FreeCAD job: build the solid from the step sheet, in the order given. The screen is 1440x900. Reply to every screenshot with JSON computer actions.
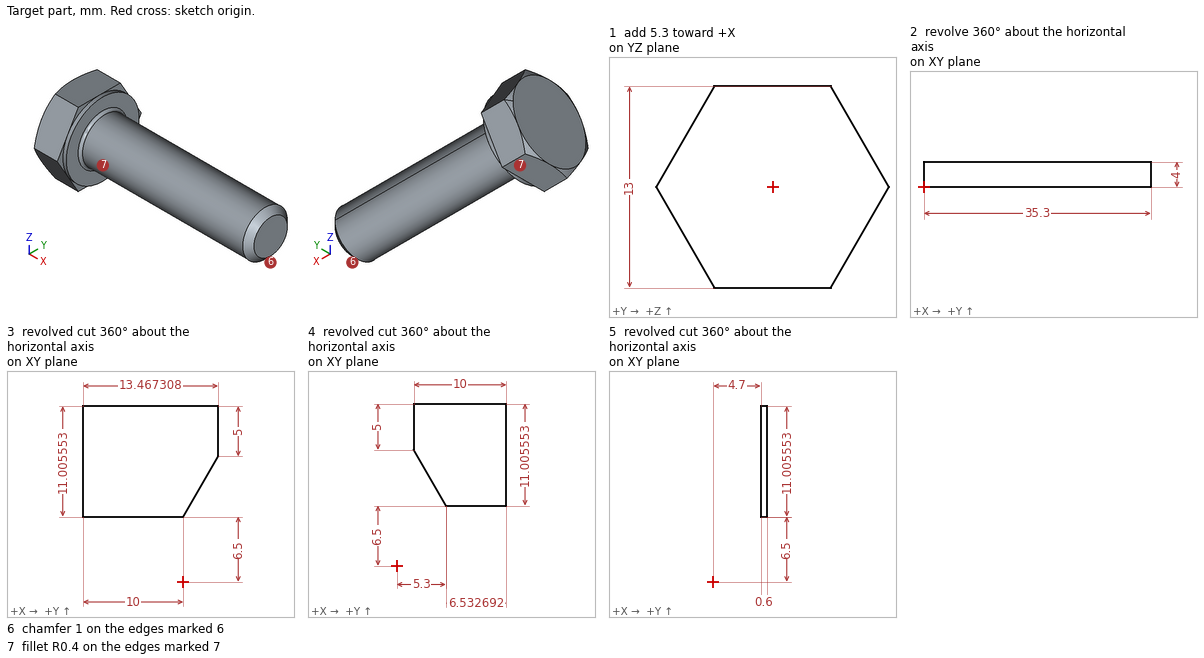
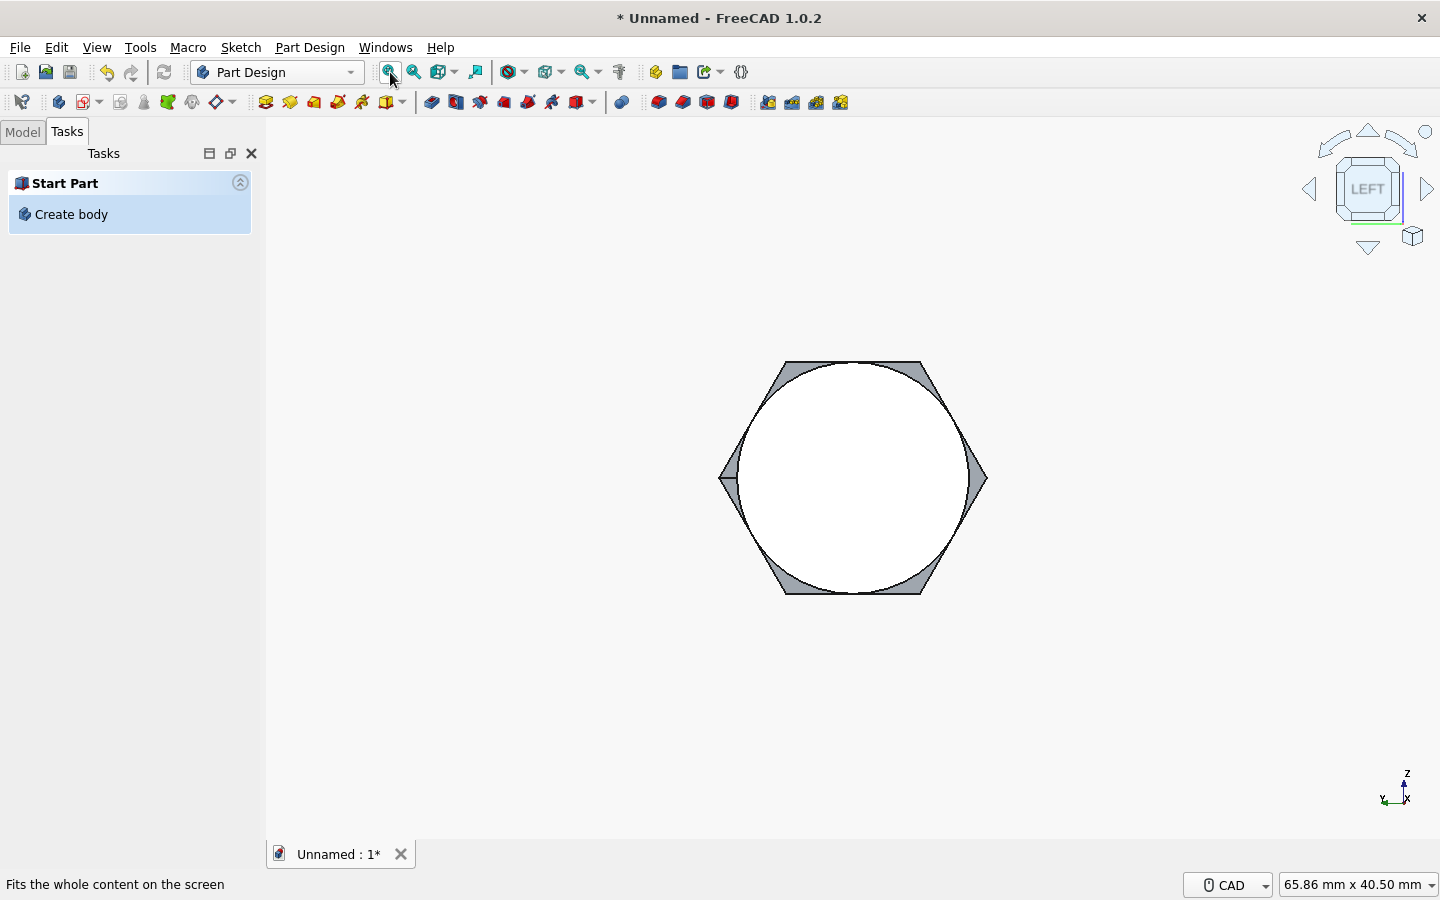
{"action": "key", "text": "v f"}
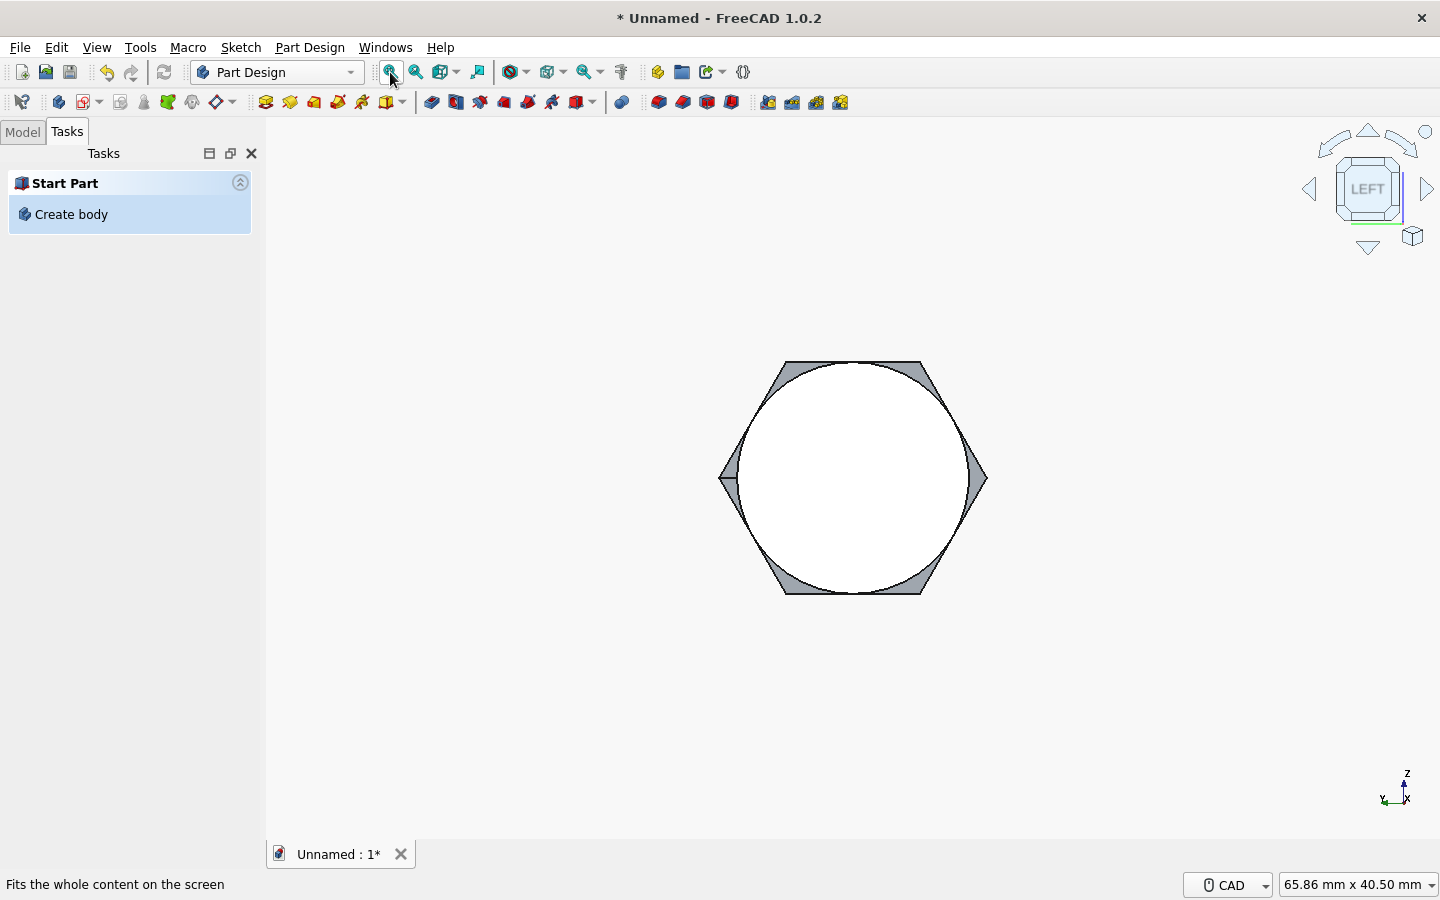
{"action": "key", "text": "v 3"}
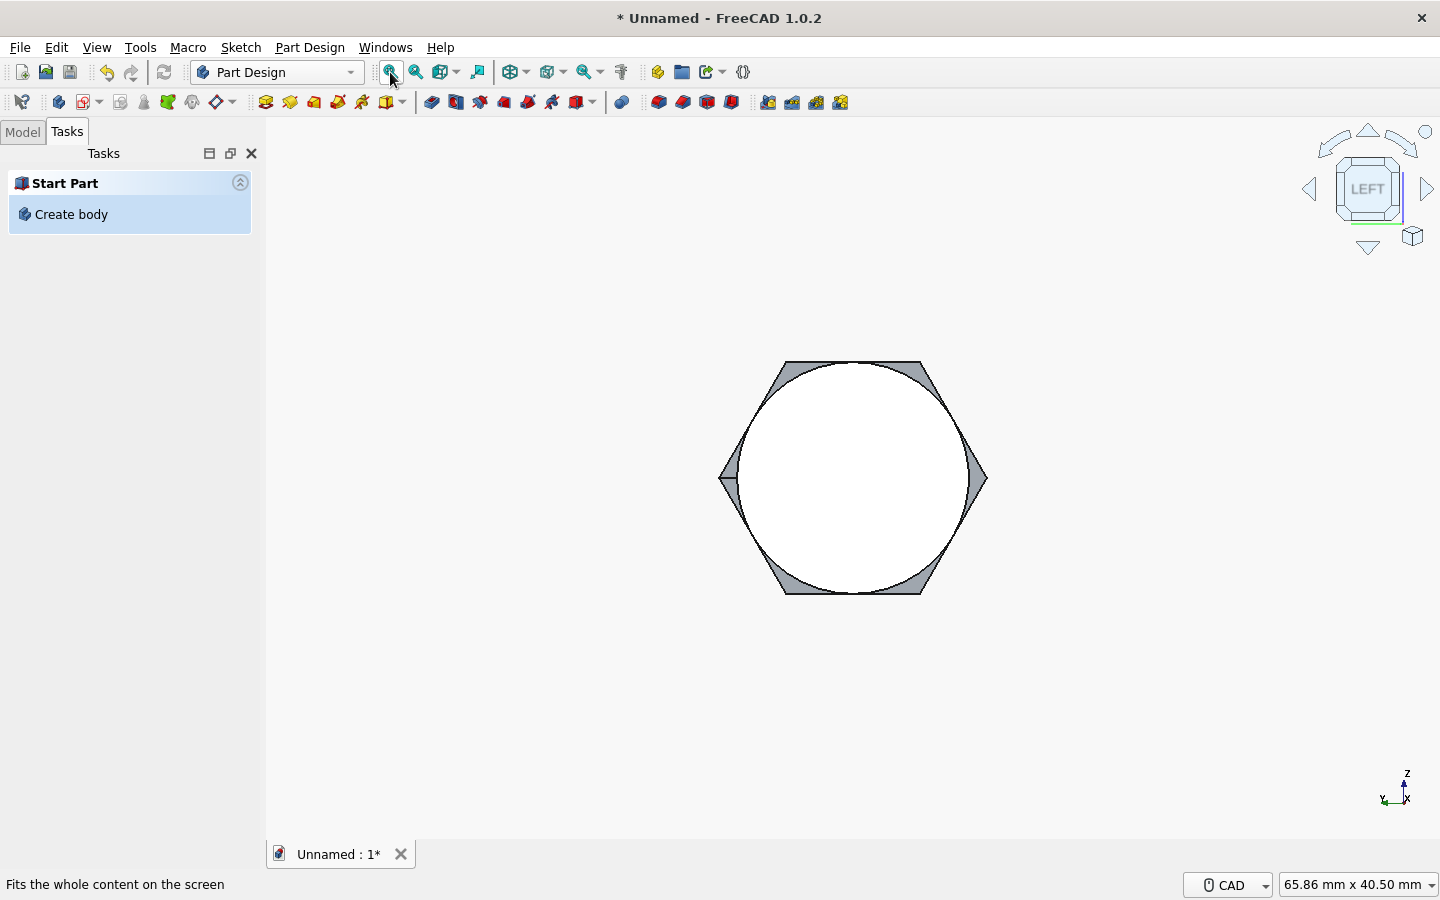
{"action": "key", "text": "0"}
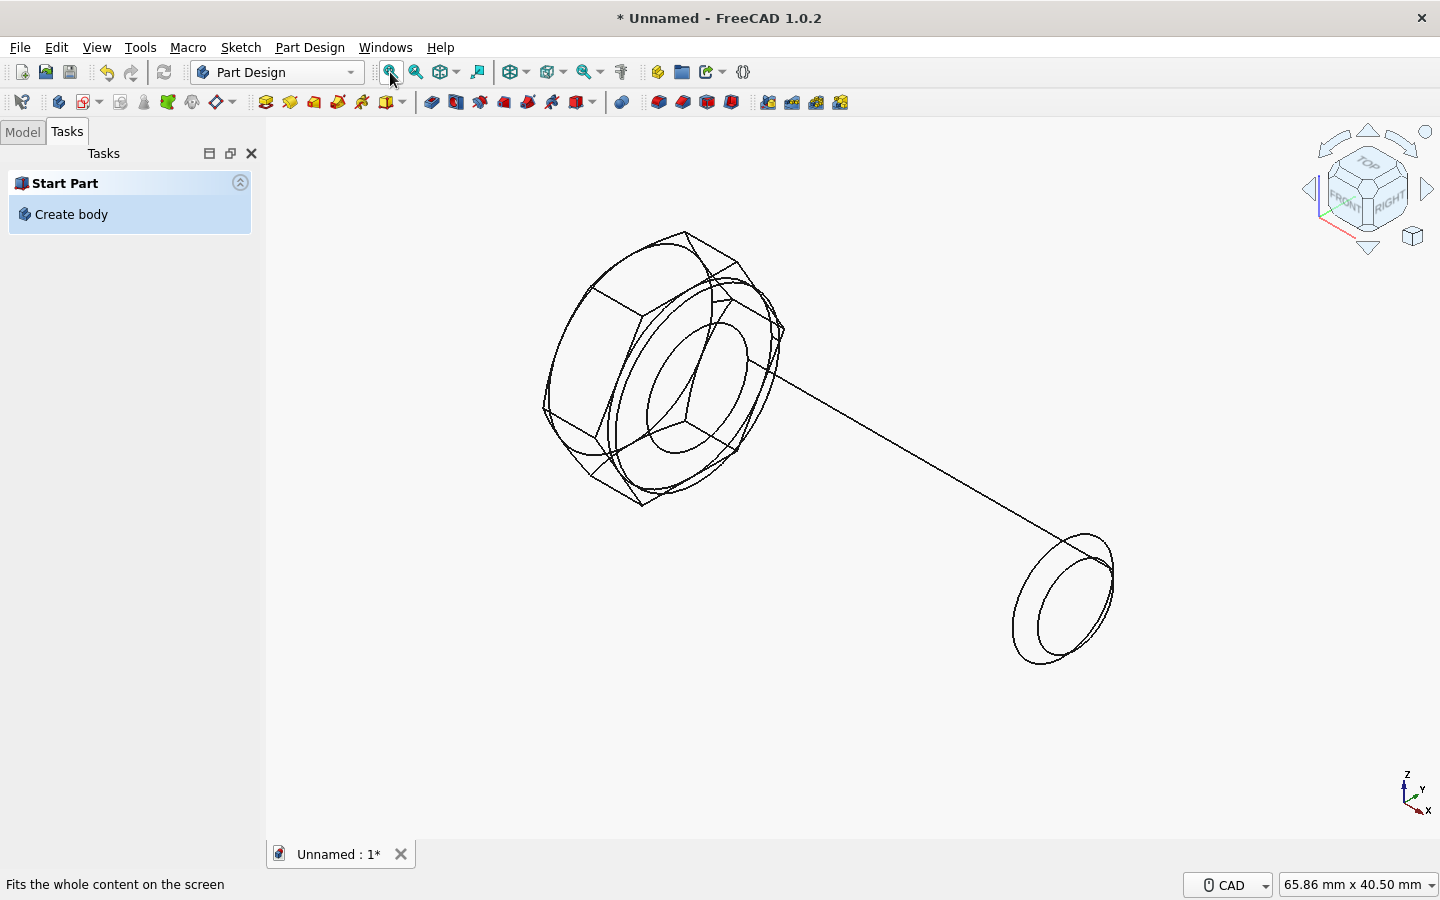
{"action": "left_click", "coordinate": [647, 416]}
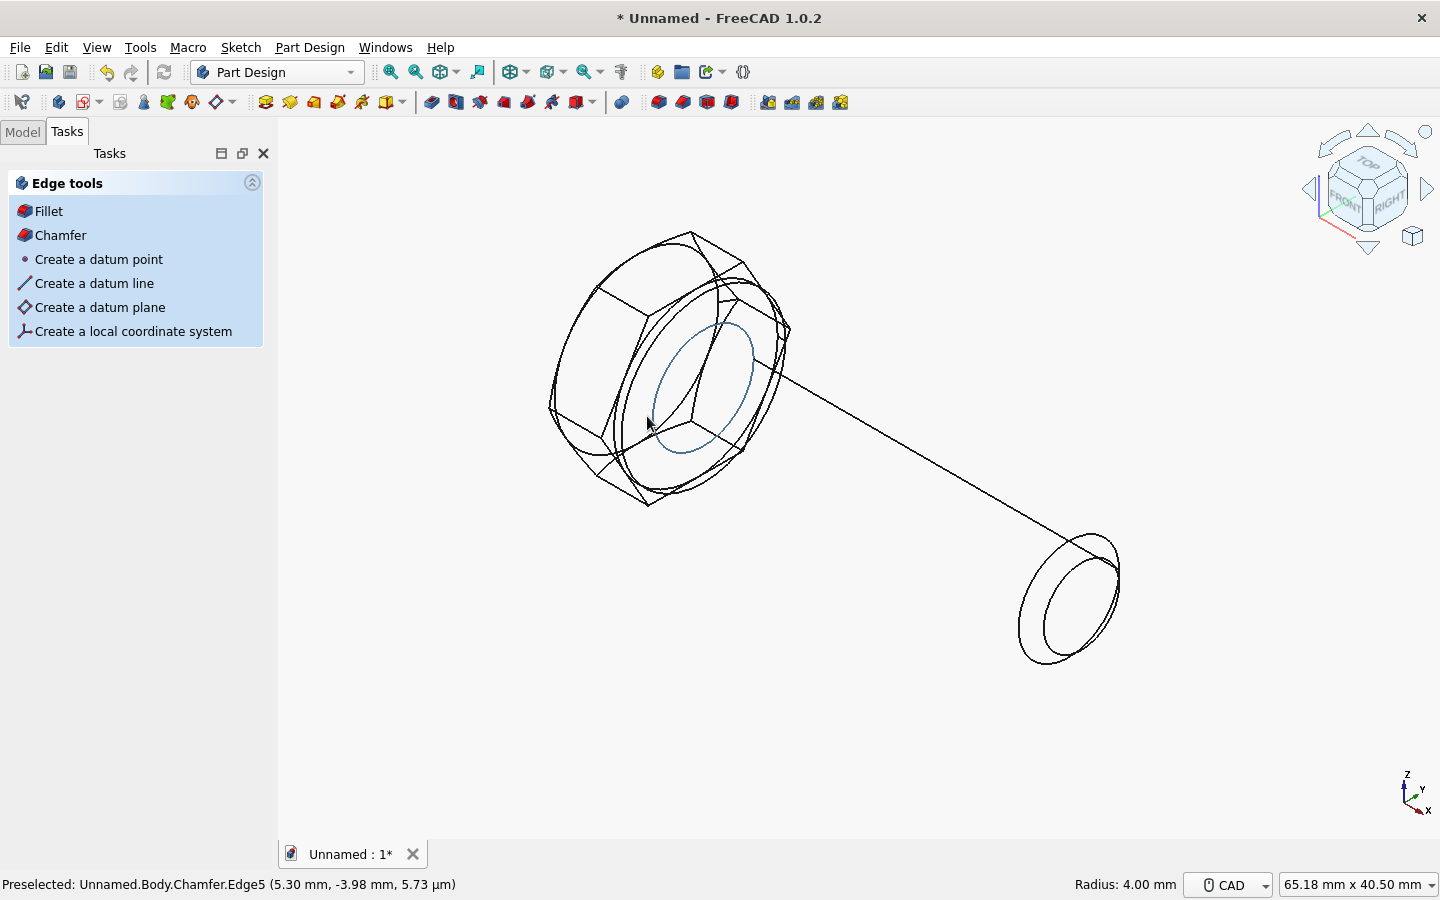
{"action": "key", "text": "v 1"}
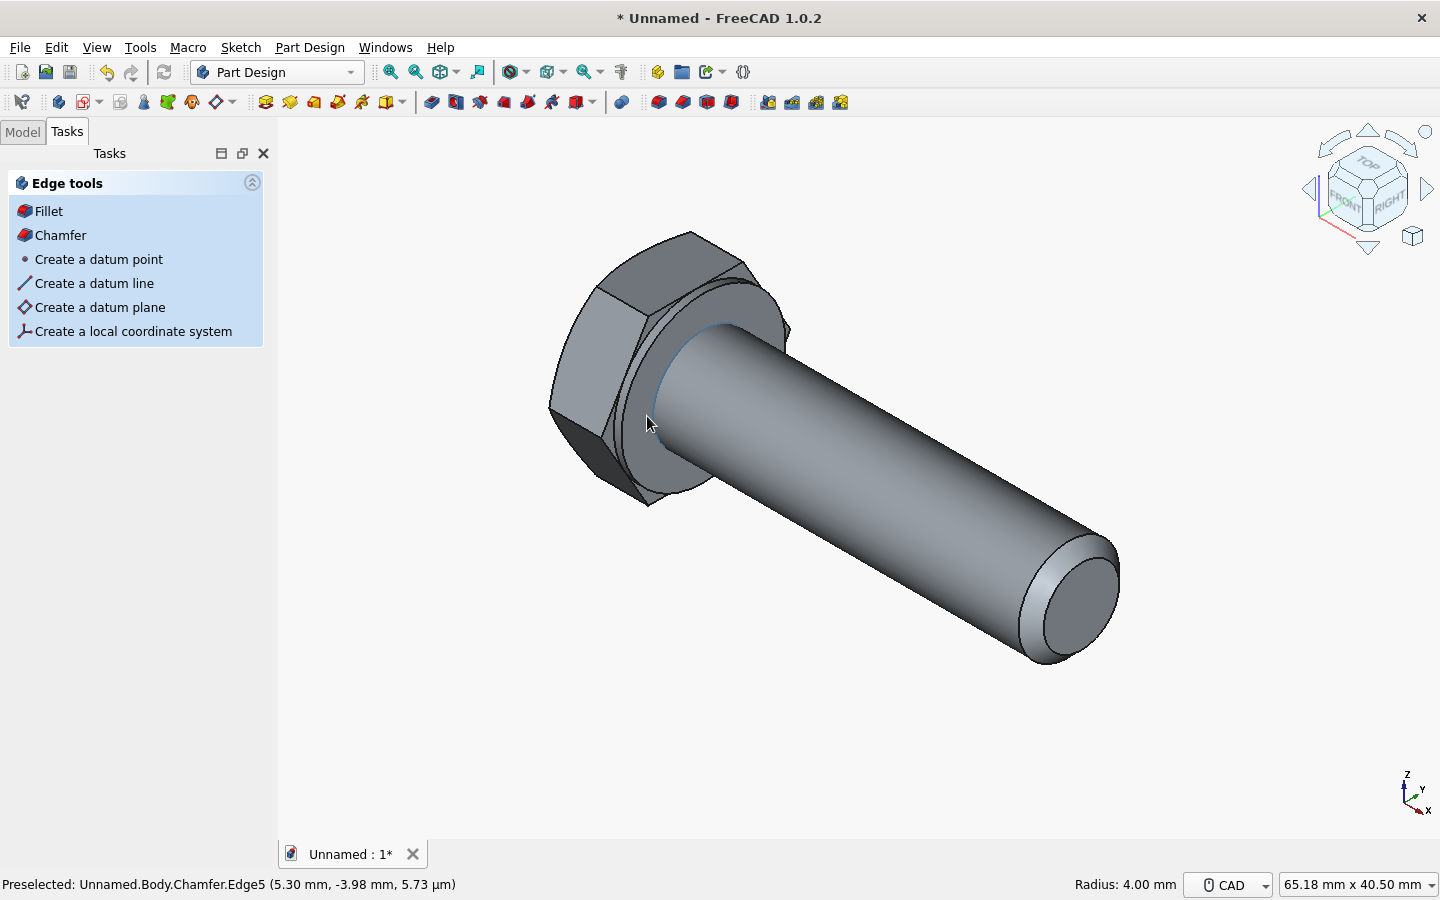
{"action": "left_click", "coordinate": [660, 102]}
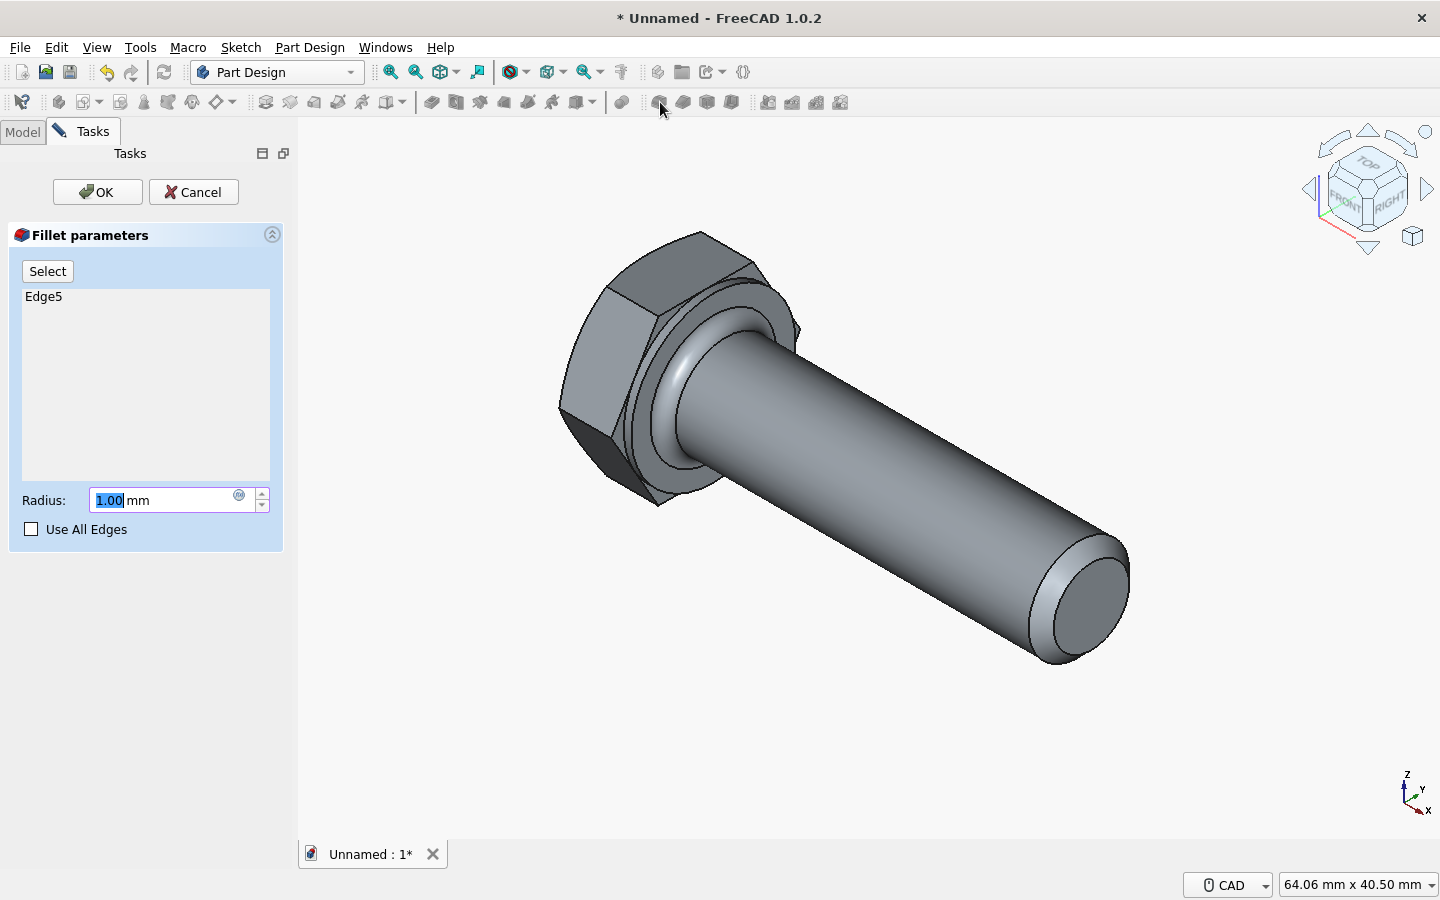
{"action": "type", "text": "0.4"}
{"action": "key", "text": "Tab"}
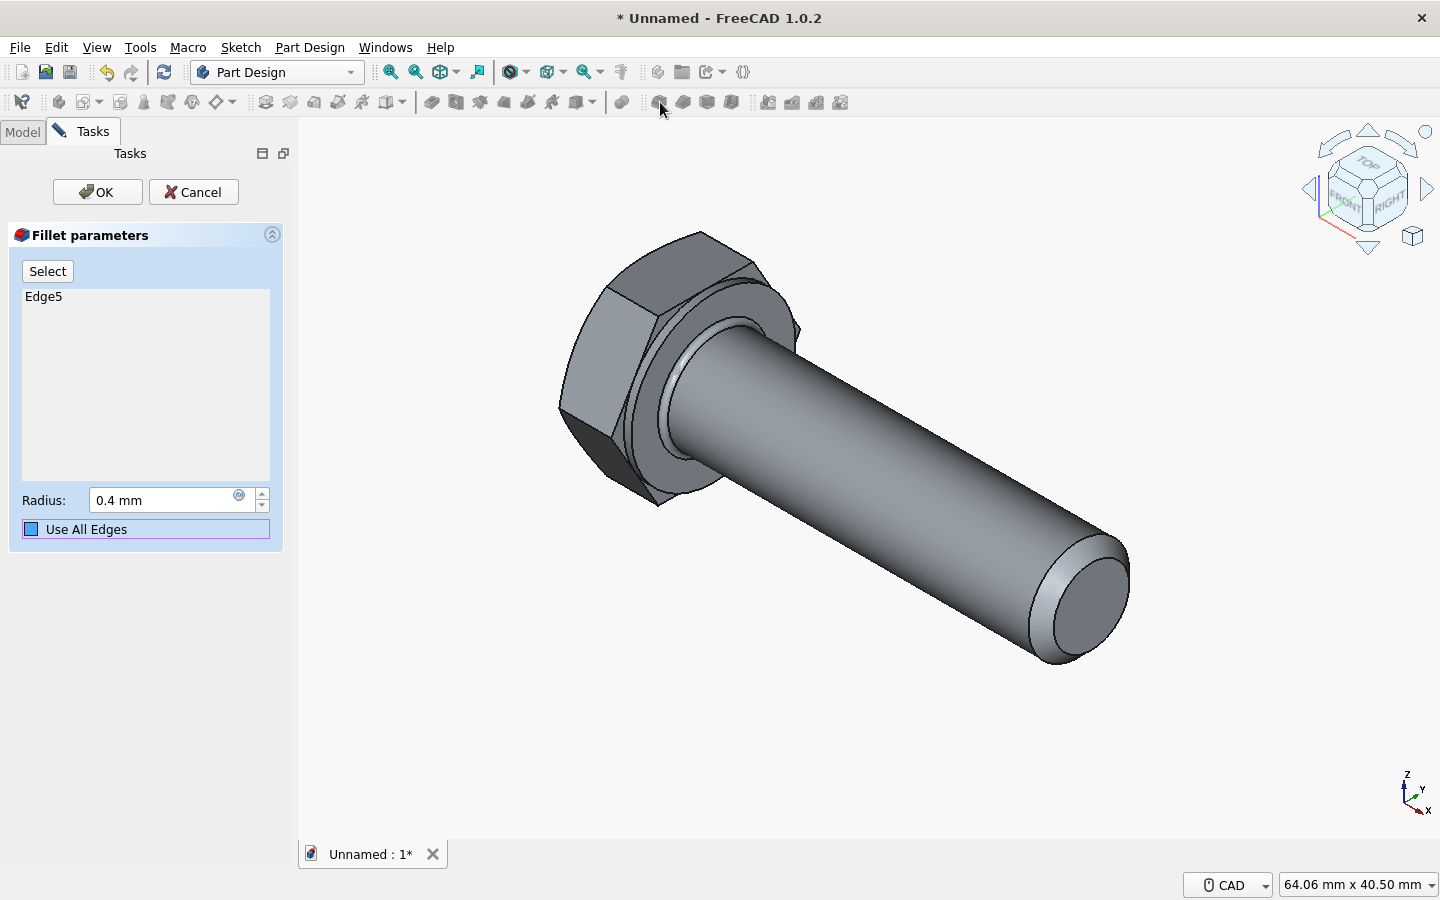
{"action": "left_click", "coordinate": [98, 192]}